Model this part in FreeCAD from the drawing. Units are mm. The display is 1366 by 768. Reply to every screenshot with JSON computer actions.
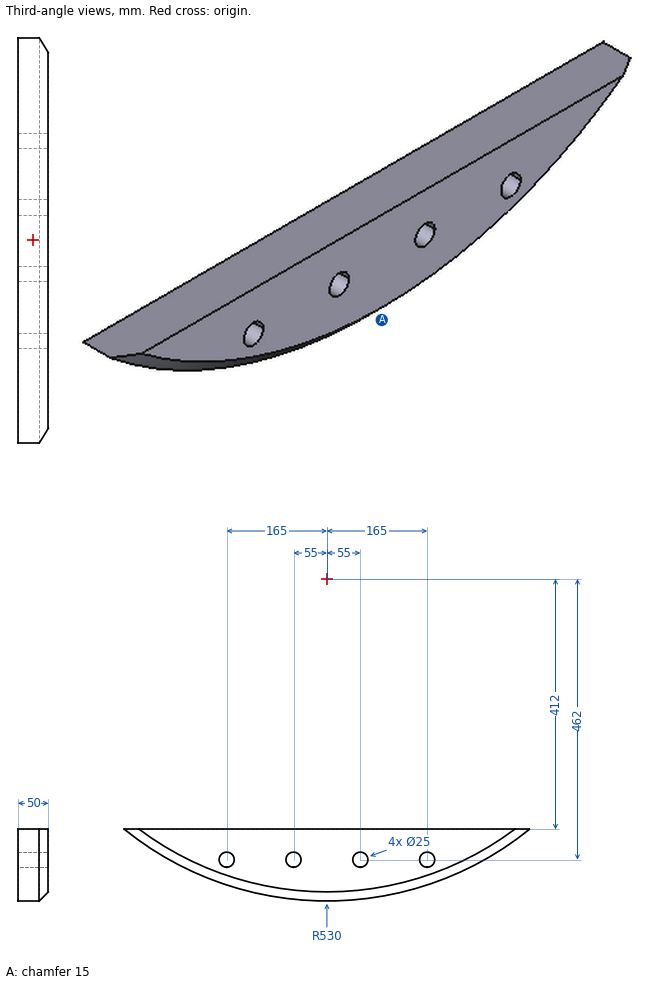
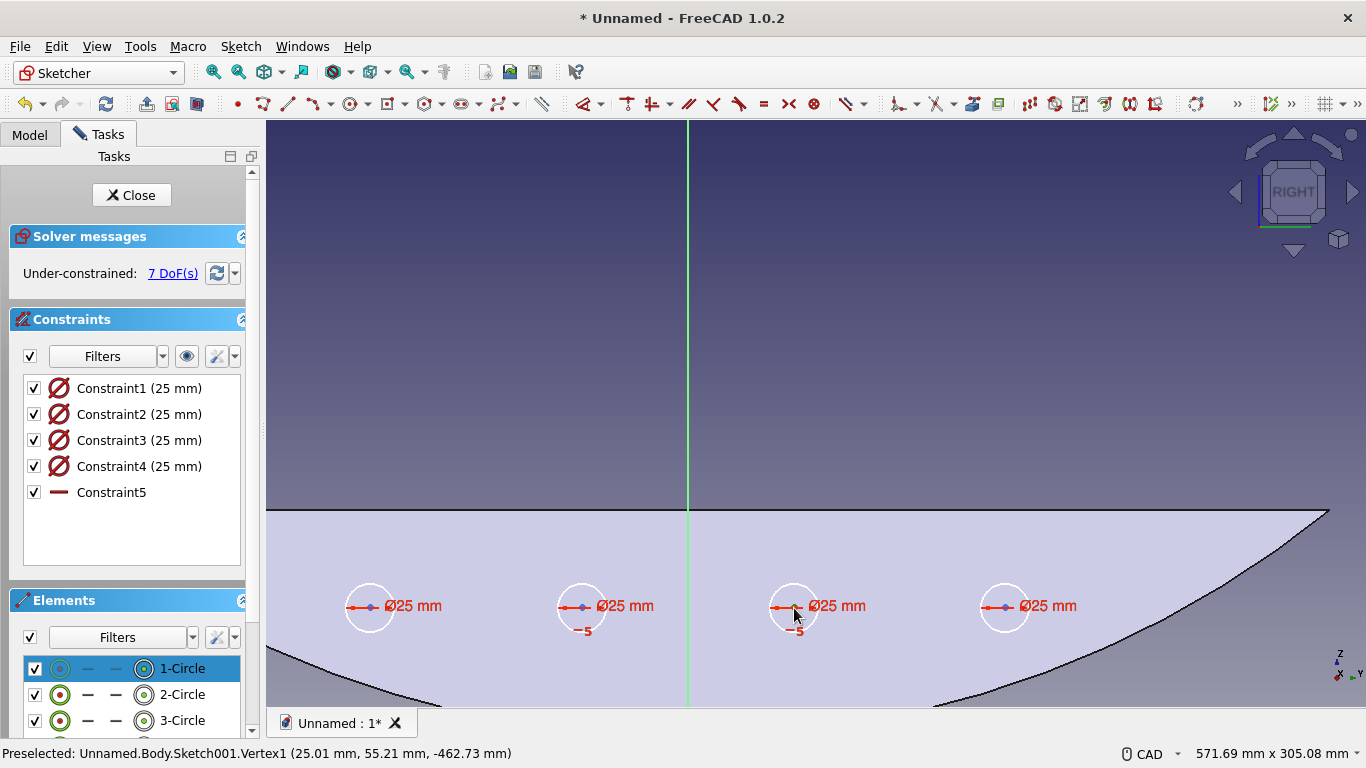
{"action": "left_click", "coordinate": [1005, 608]}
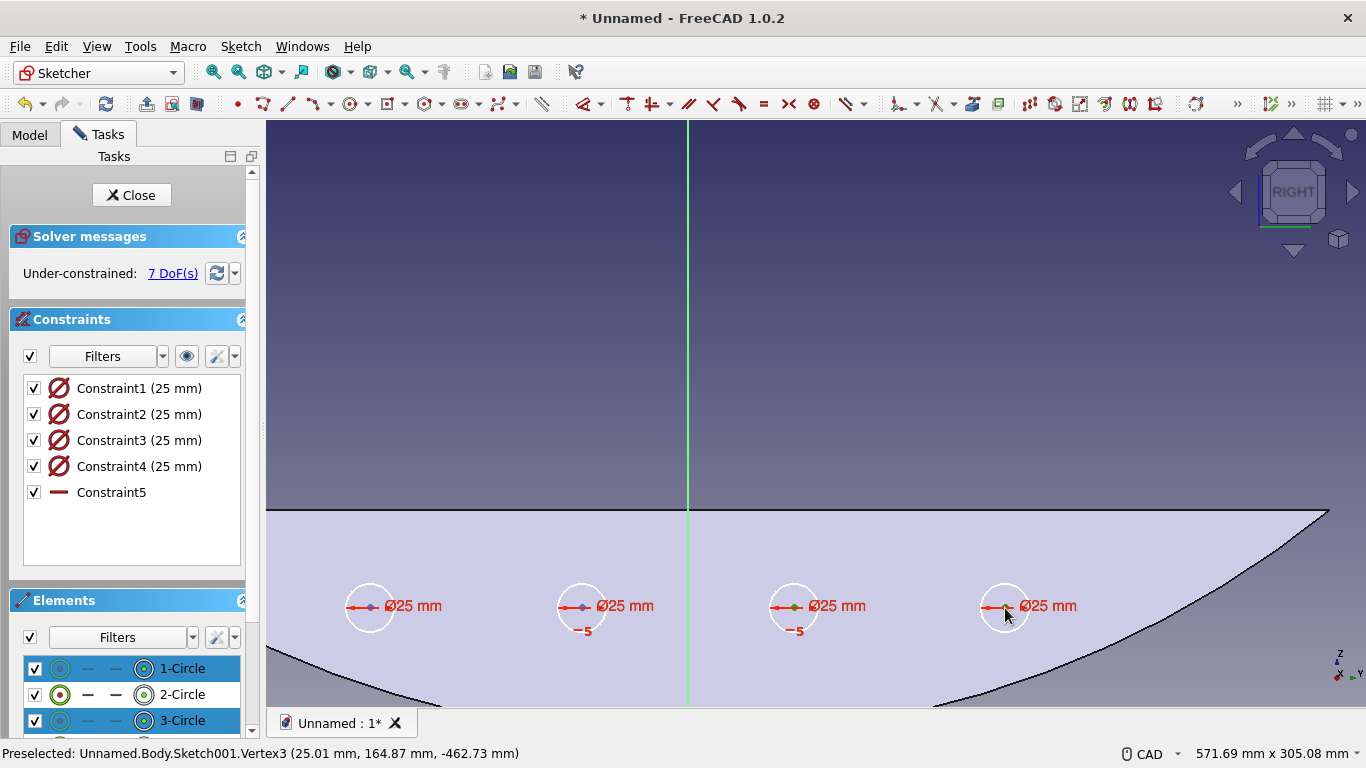
{"action": "left_click", "coordinate": [670, 104]}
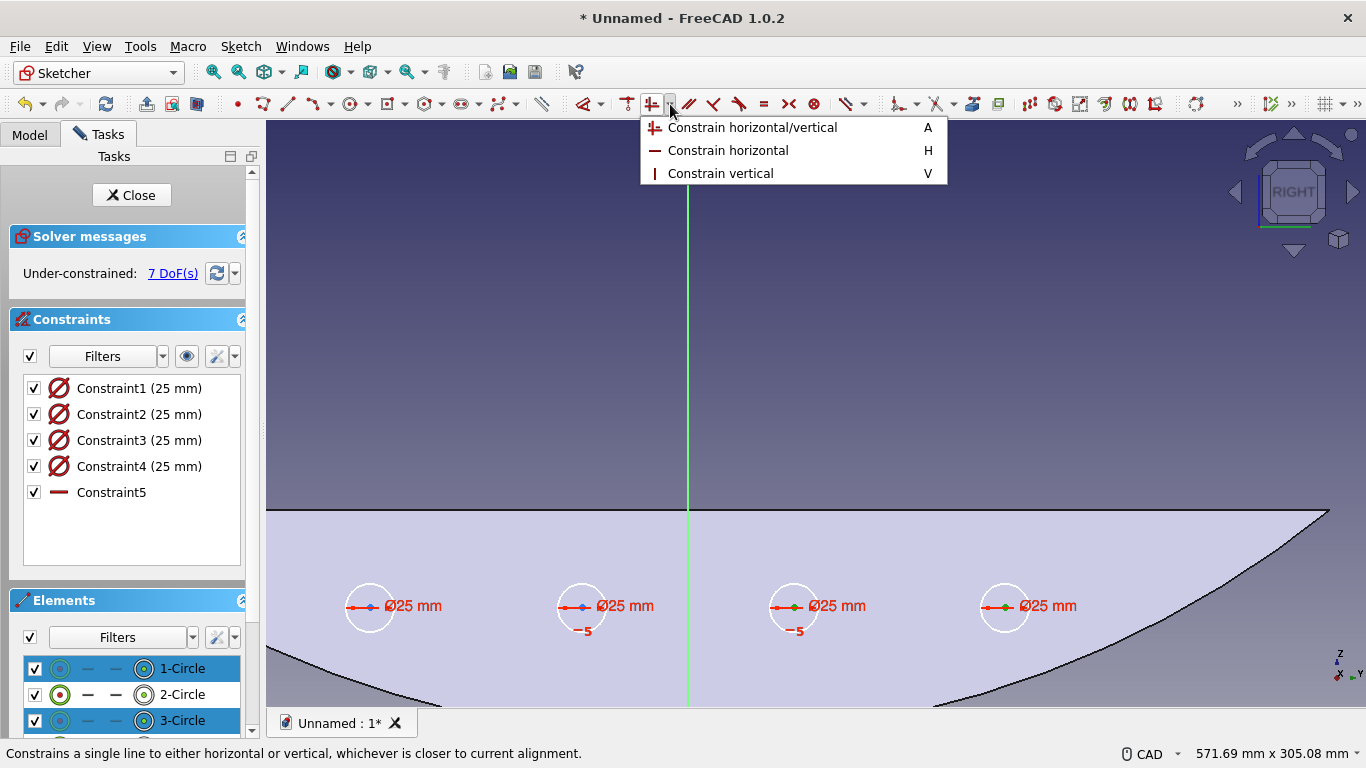
{"action": "left_click", "coordinate": [794, 150]}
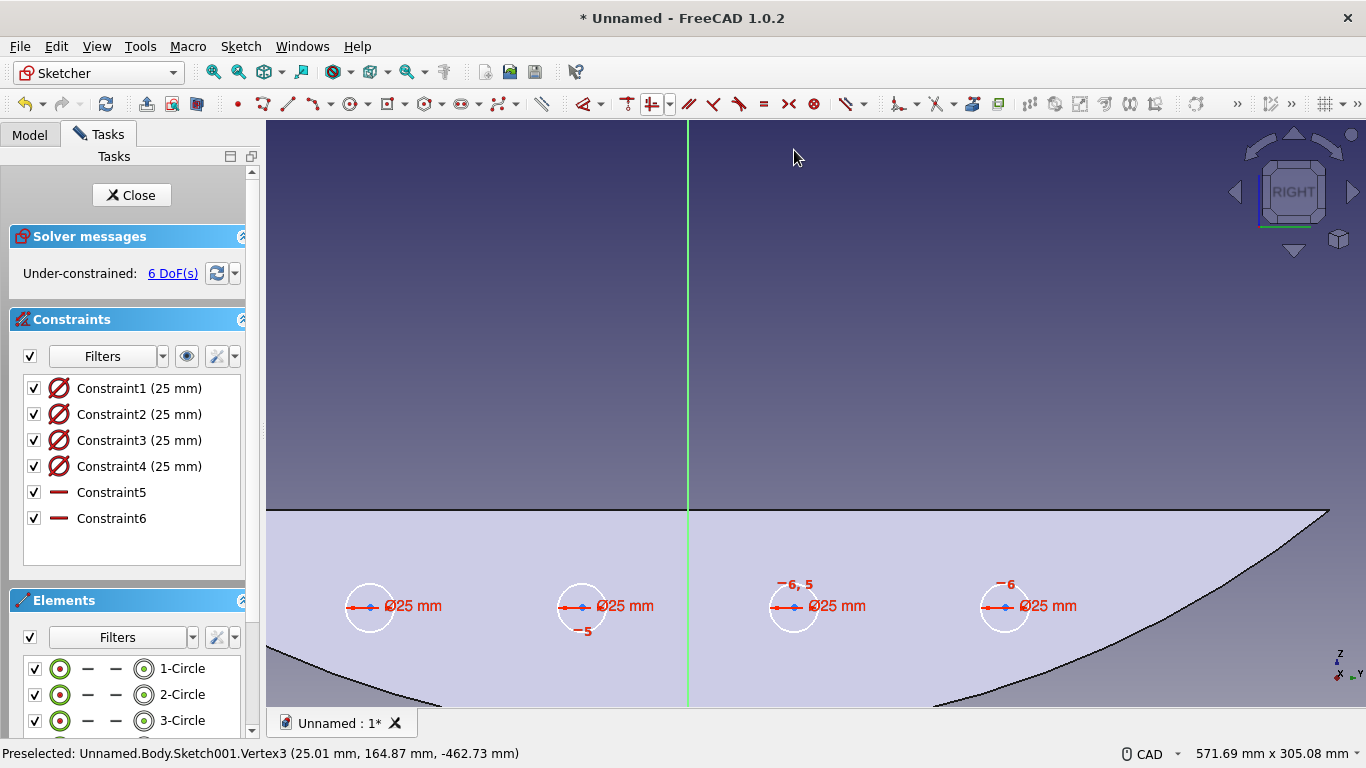
{"action": "left_click", "coordinate": [582, 608]}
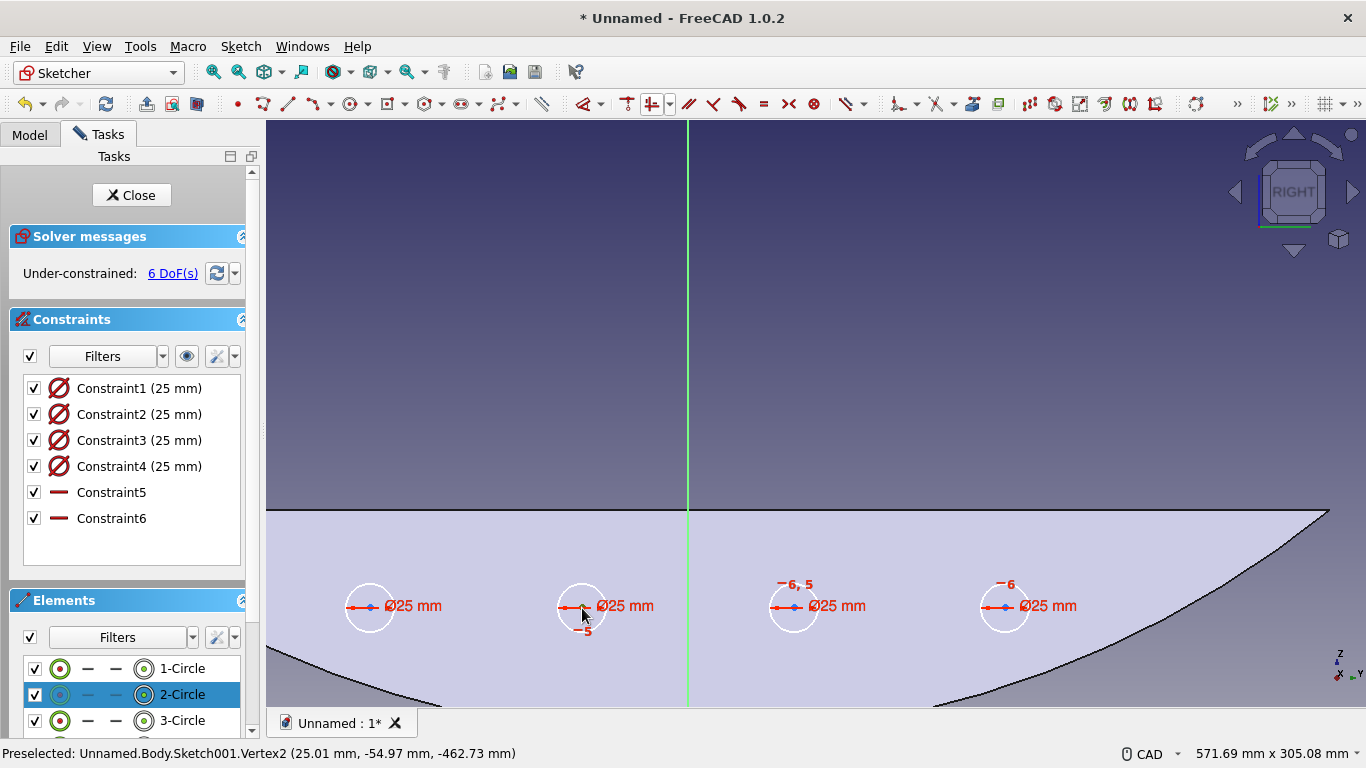
{"action": "left_click", "coordinate": [370, 608]}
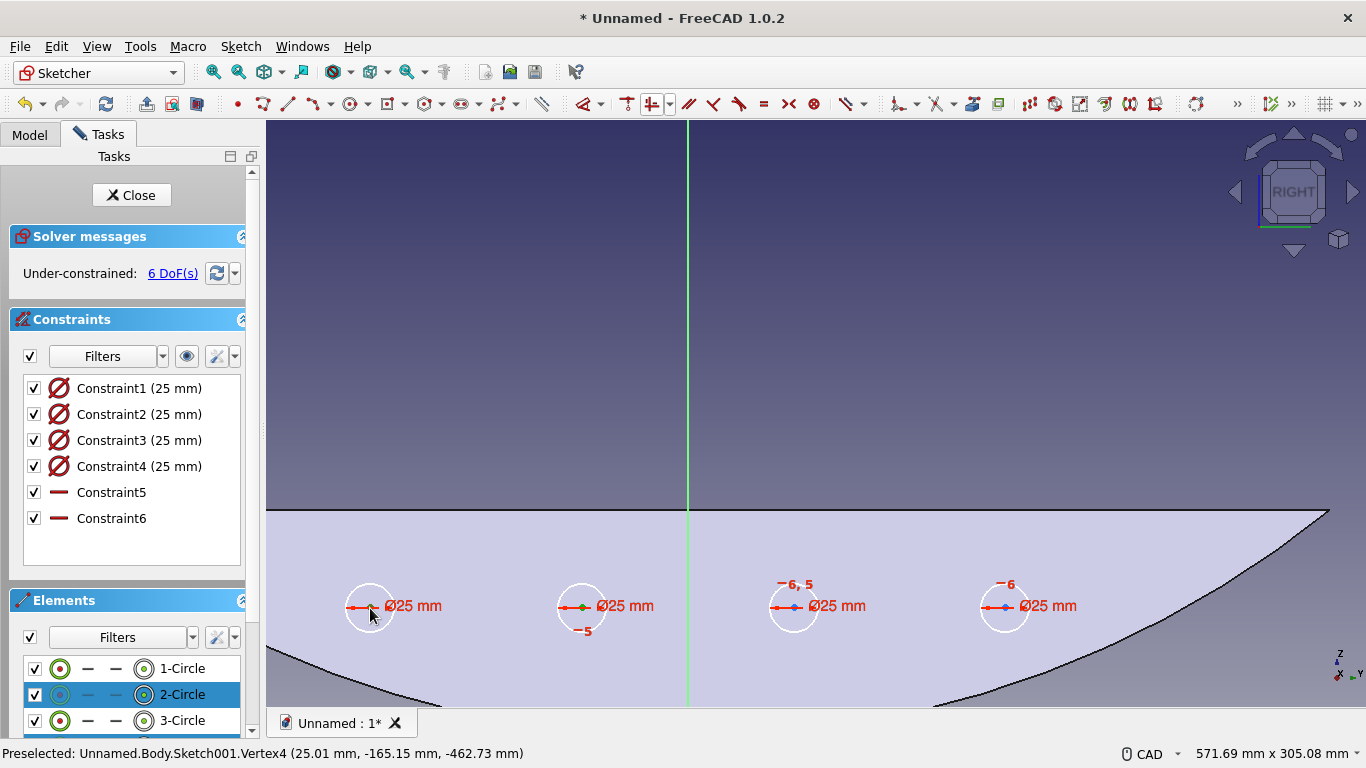
{"action": "left_click", "coordinate": [670, 104]}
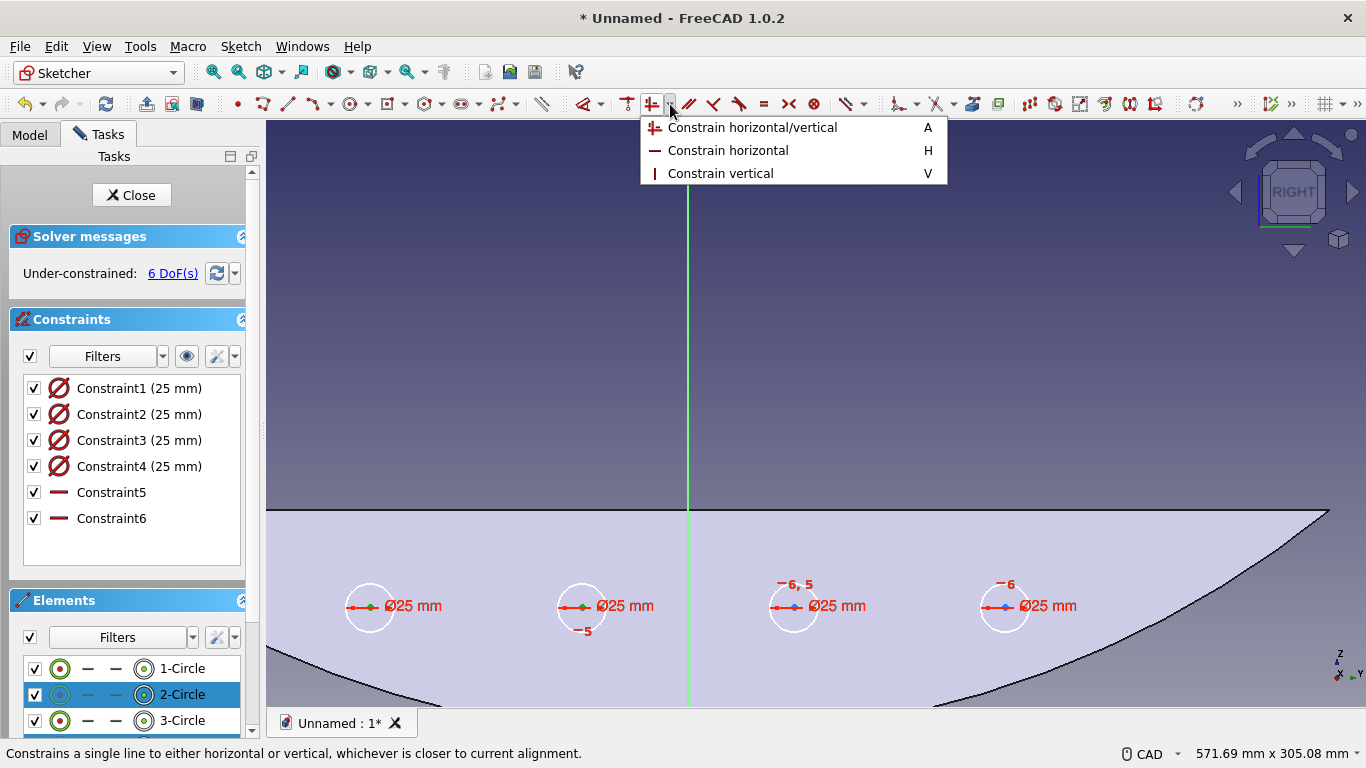
{"action": "left_click", "coordinate": [794, 150]}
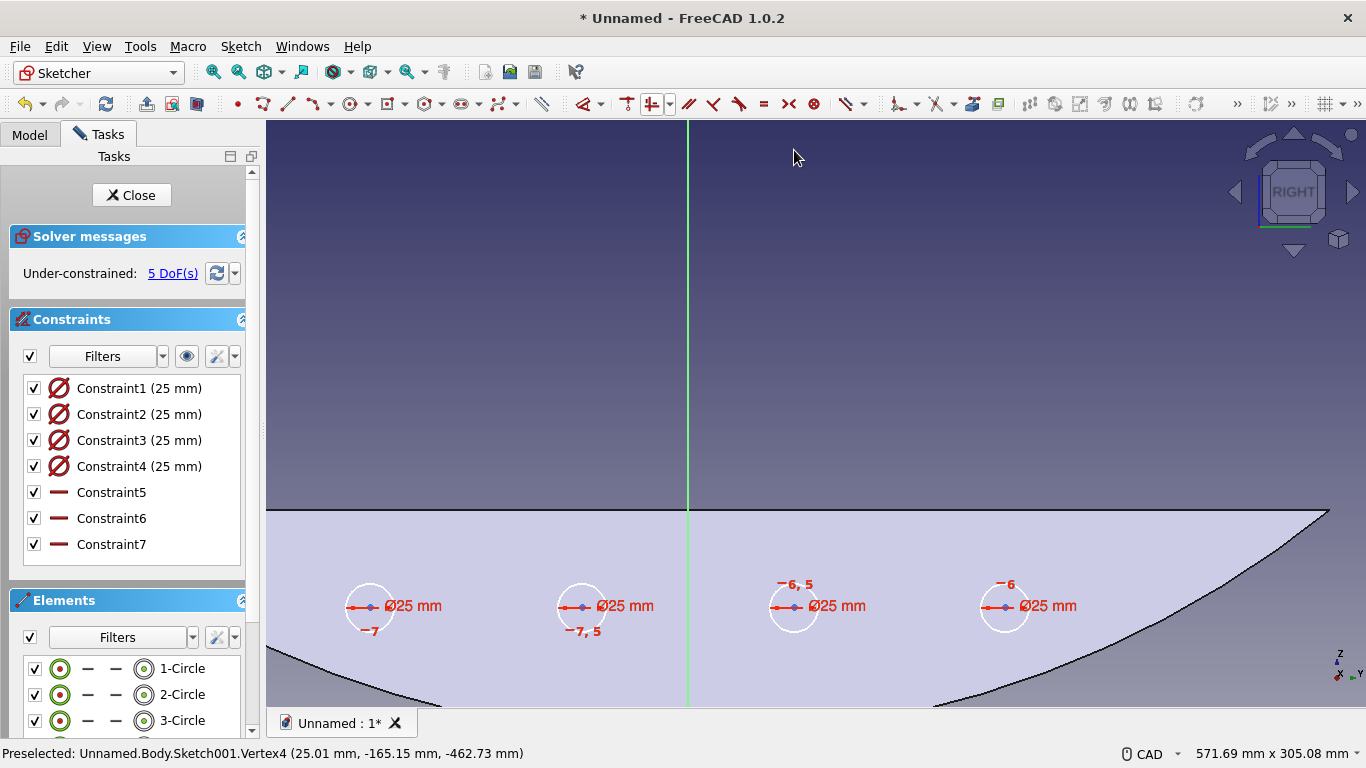
{"action": "left_click", "coordinate": [582, 104]}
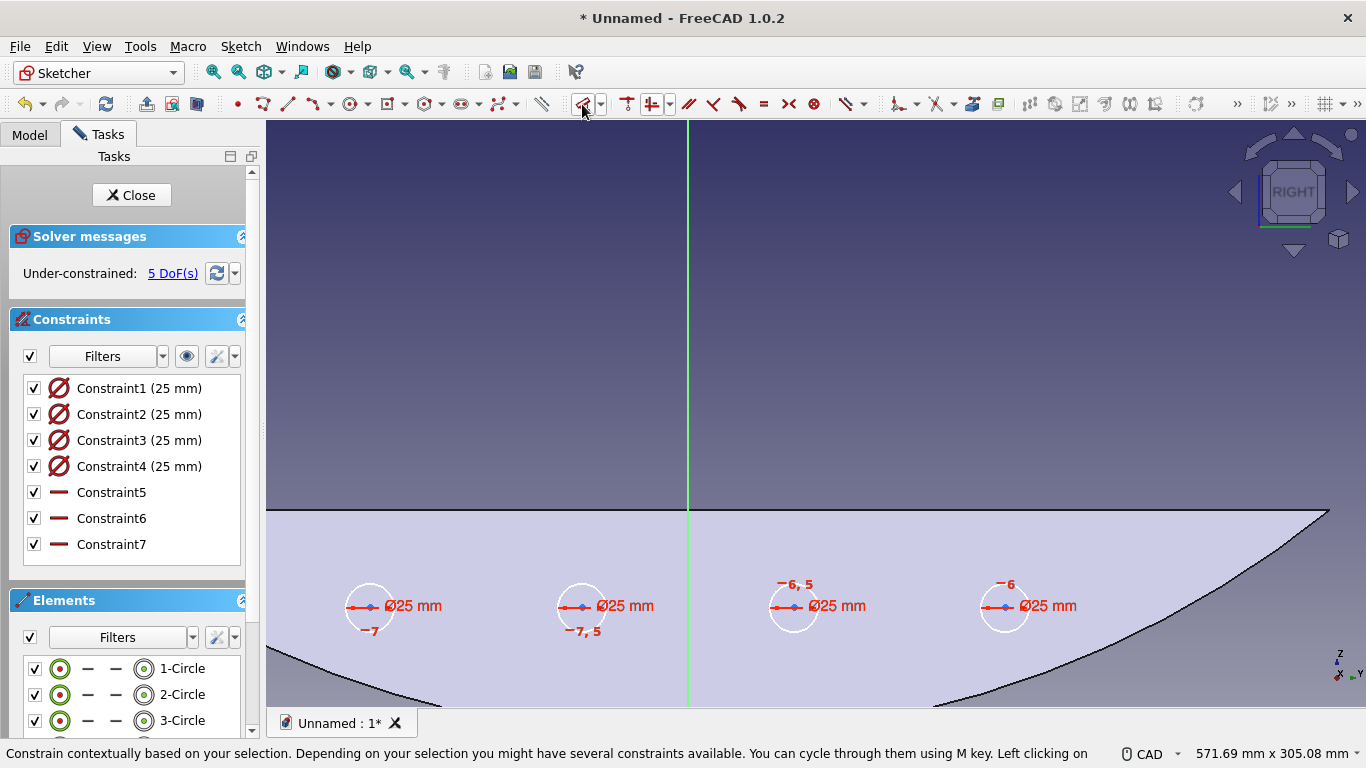
{"action": "left_click", "coordinate": [794, 608]}
{"action": "left_click", "coordinate": [741, 642]}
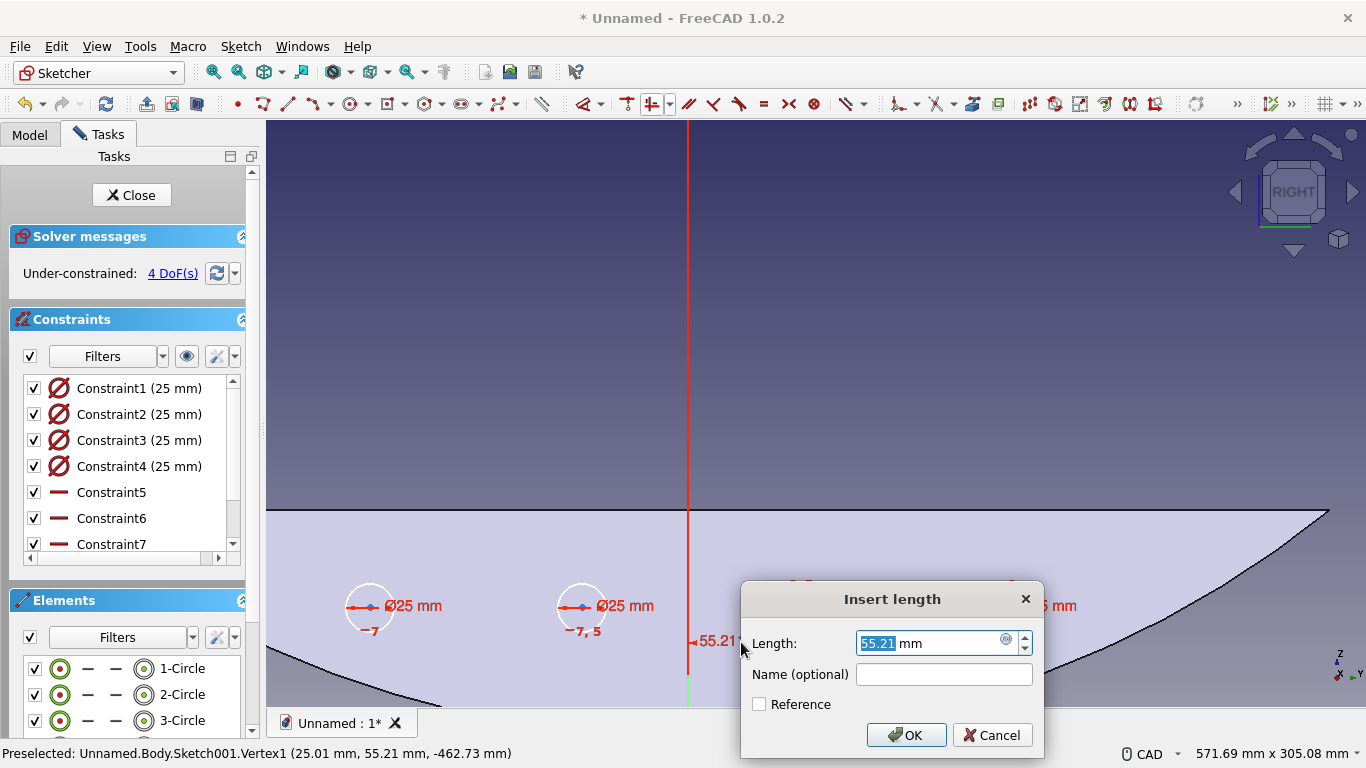
{"action": "type", "text": "55"}
{"action": "key", "text": "Return"}